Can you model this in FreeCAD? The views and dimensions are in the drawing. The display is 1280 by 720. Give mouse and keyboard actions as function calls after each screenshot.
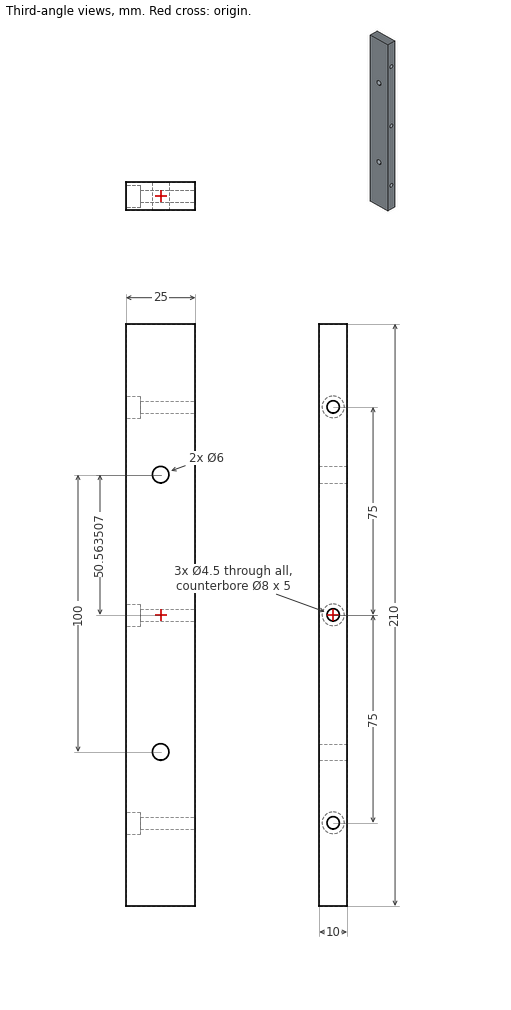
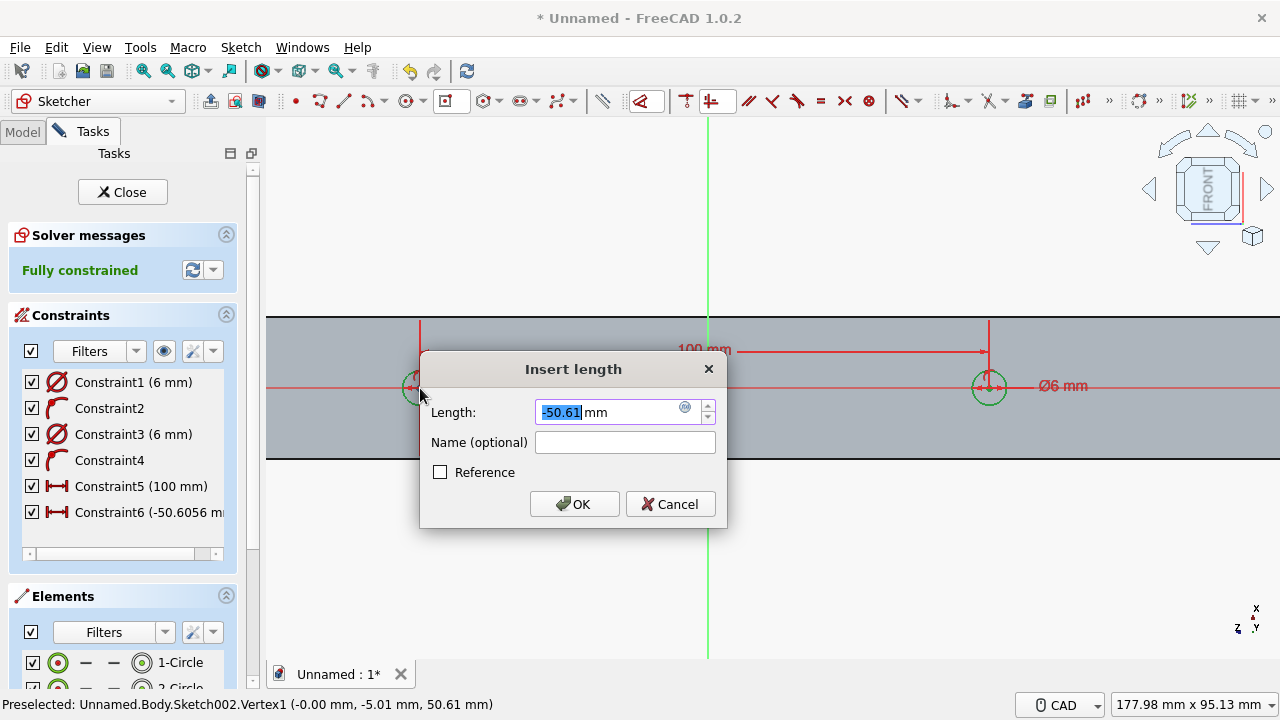
text(-50.563507)
key(Return)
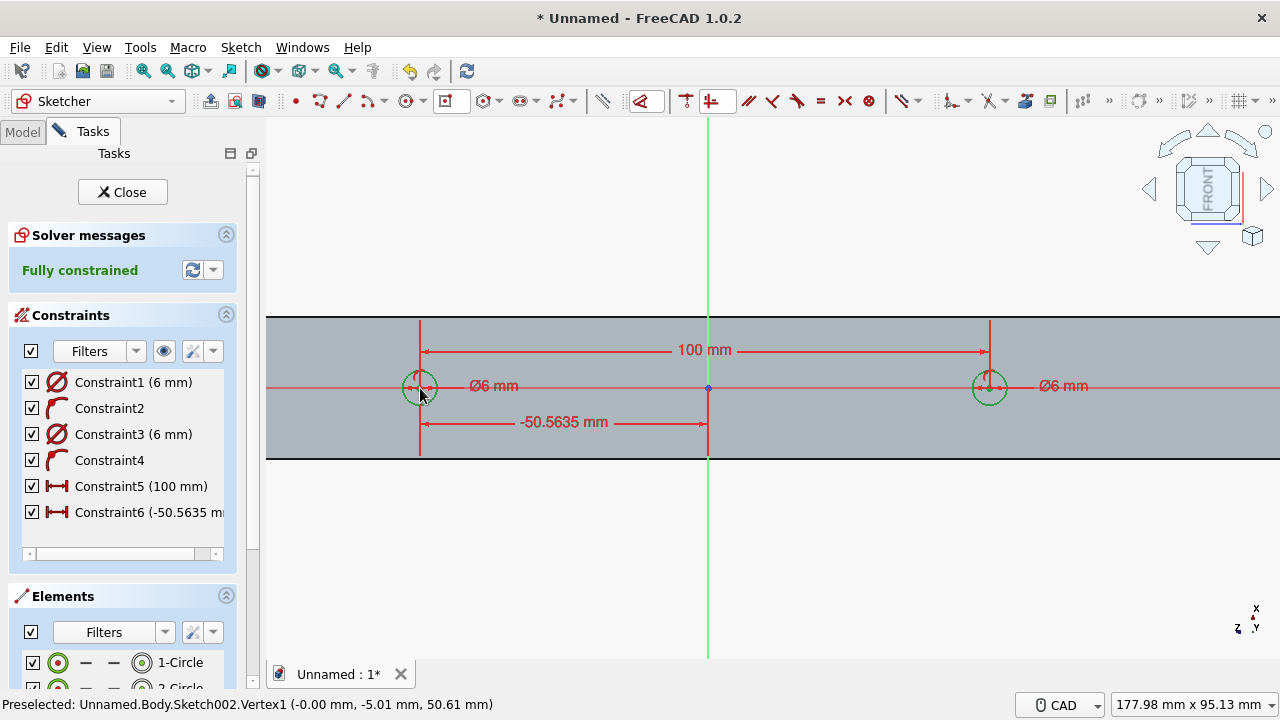
click(123, 192)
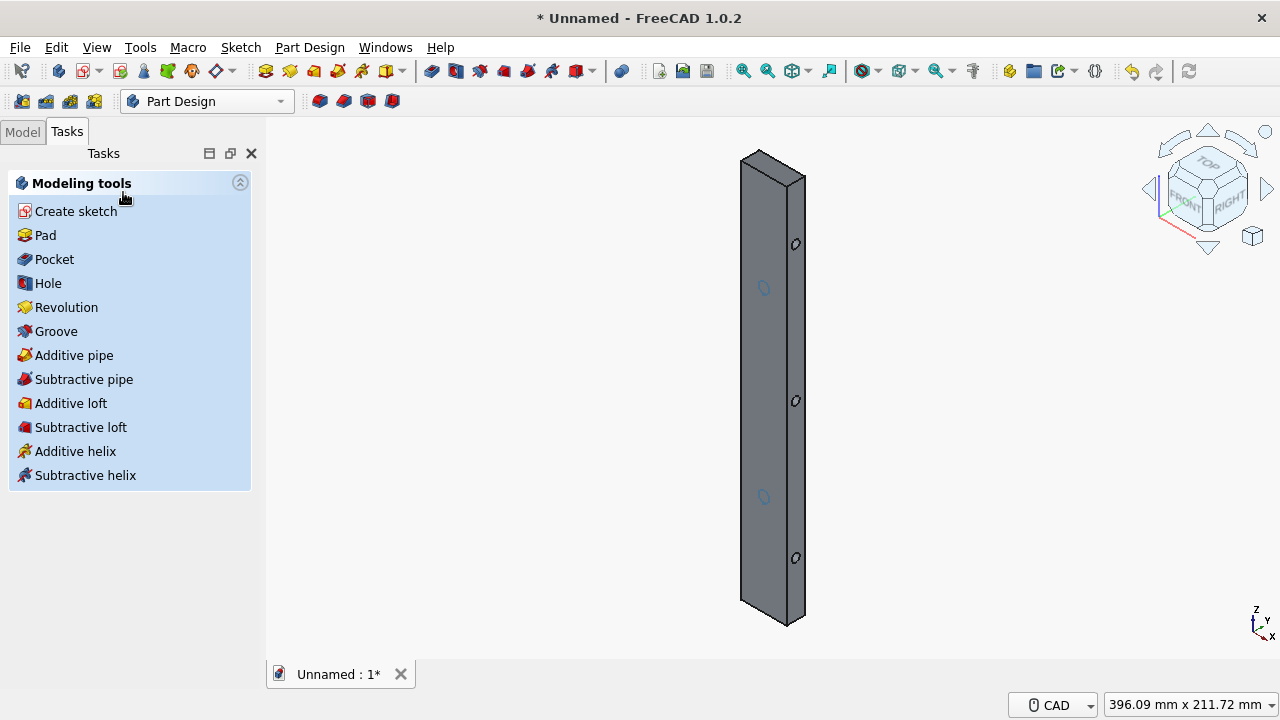
click(432, 72)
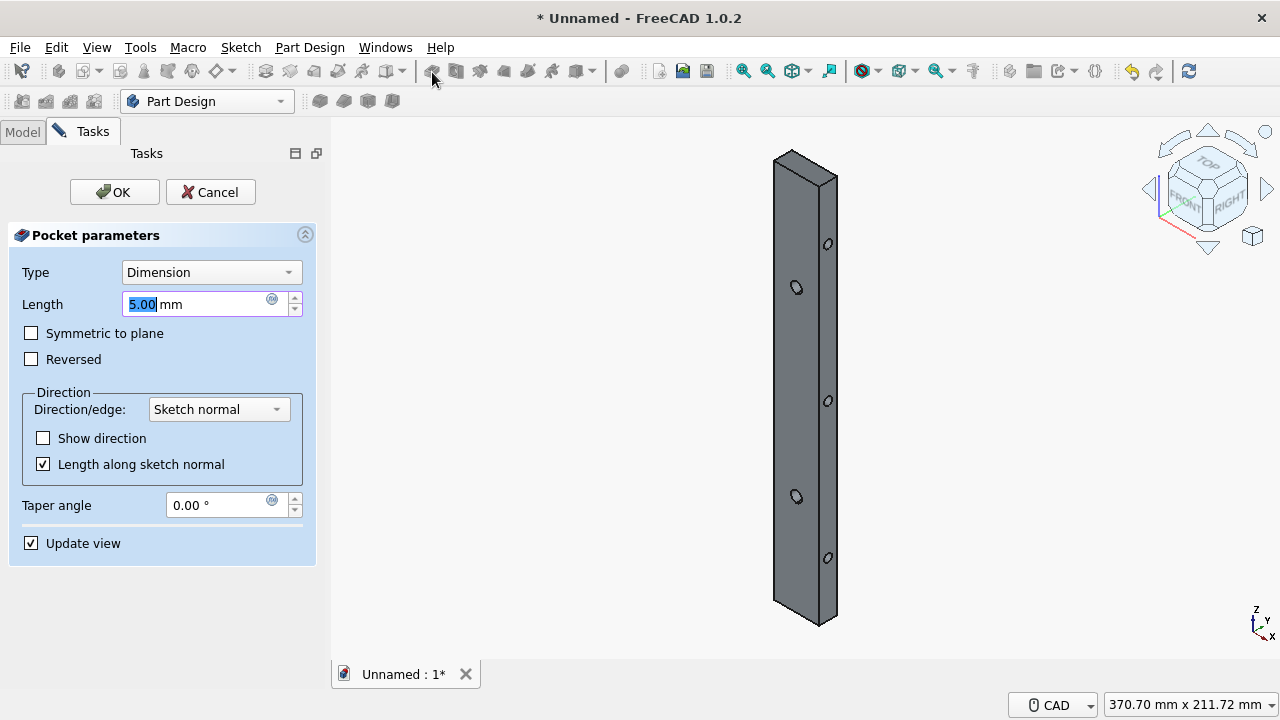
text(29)
key(Tab)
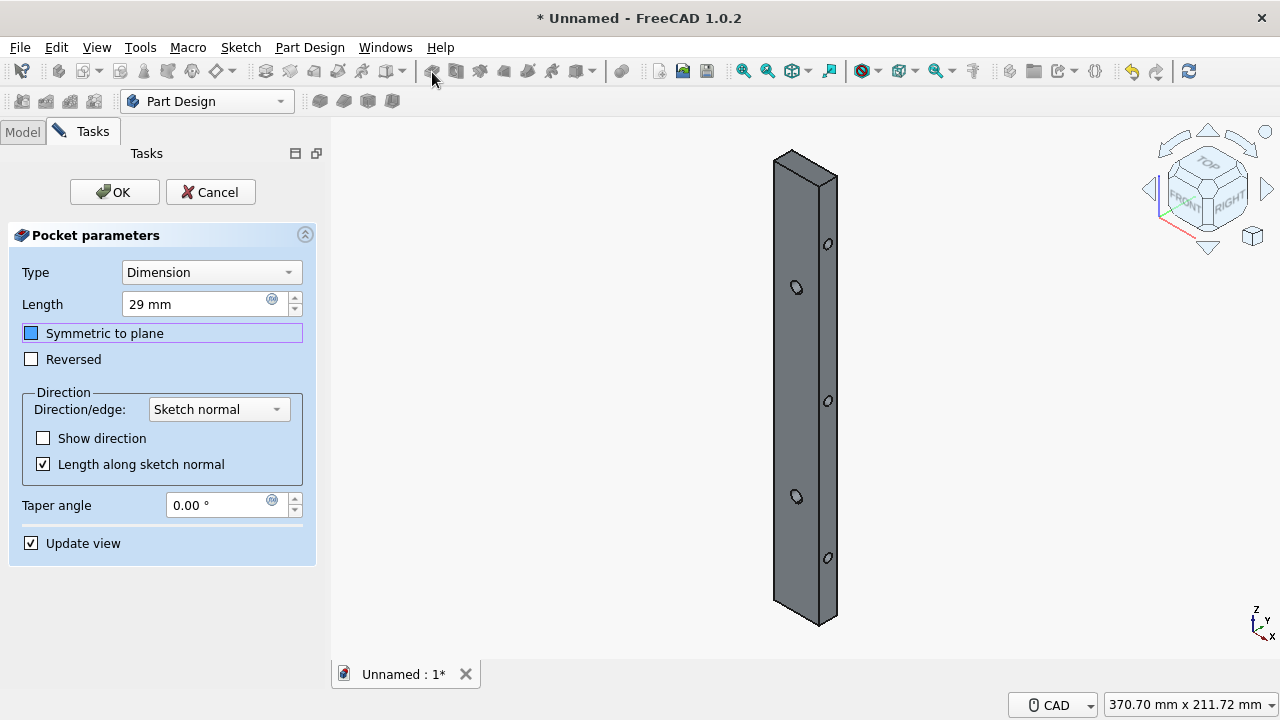
click(115, 192)